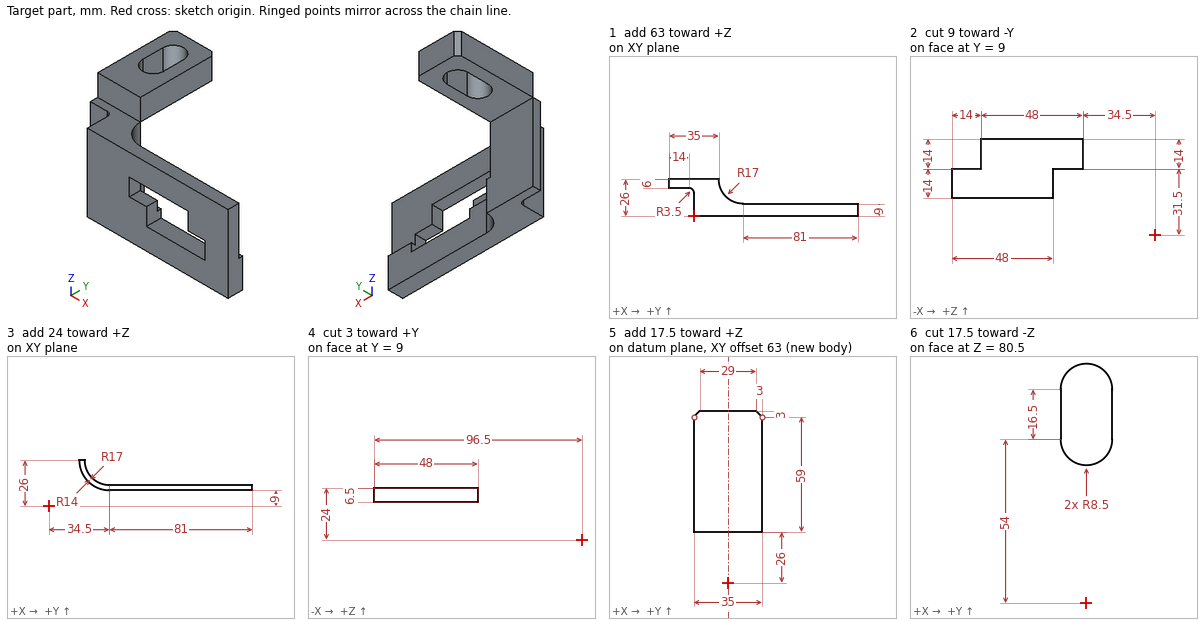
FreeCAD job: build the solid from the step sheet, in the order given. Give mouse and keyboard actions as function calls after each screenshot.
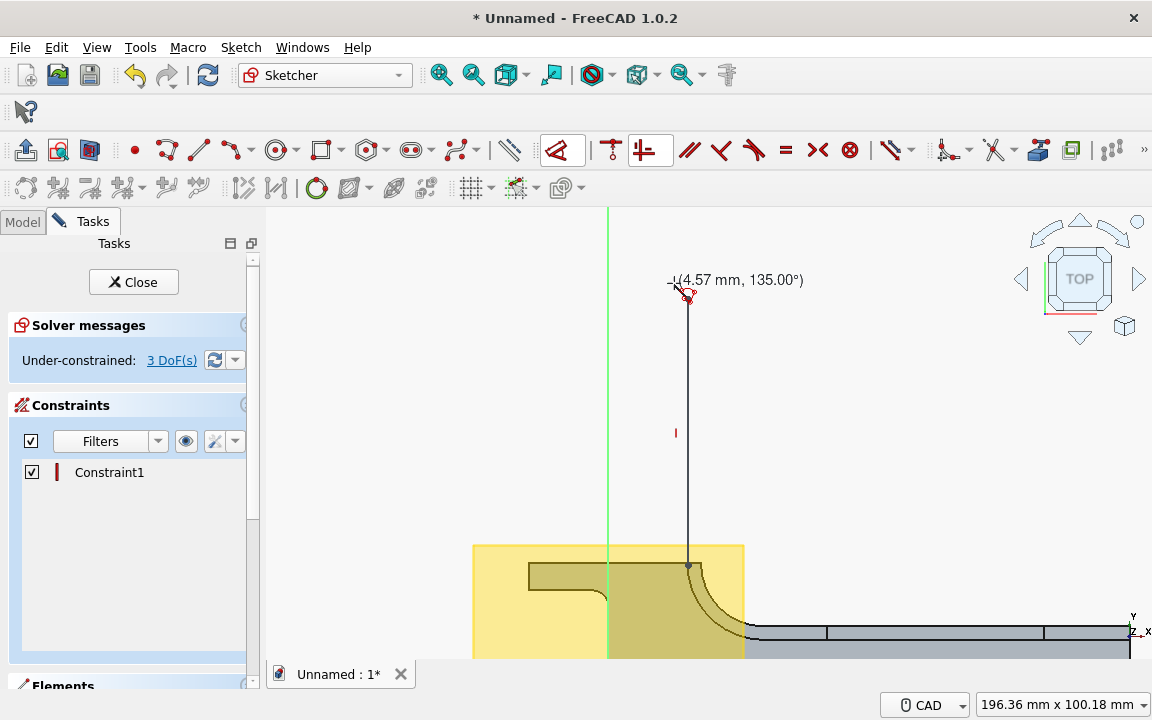
click(674, 283)
click(543, 283)
click(529, 297)
click(529, 563)
click(688, 565)
key(Escape)
key(Escape)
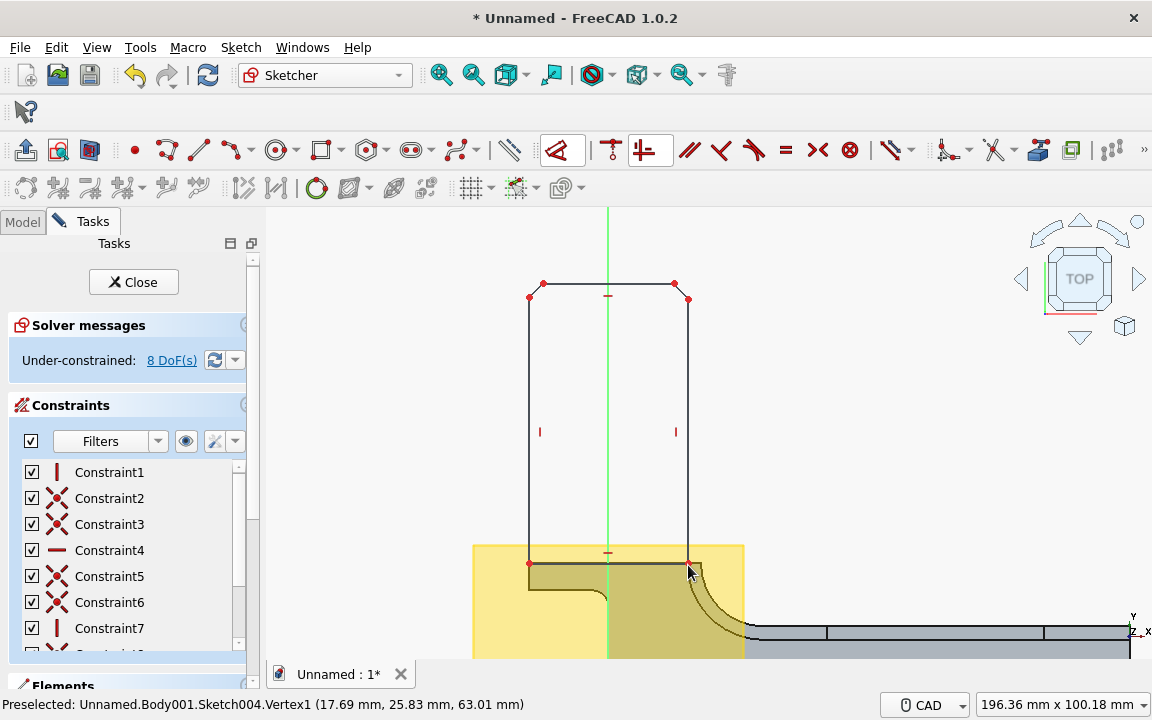
click(688, 299)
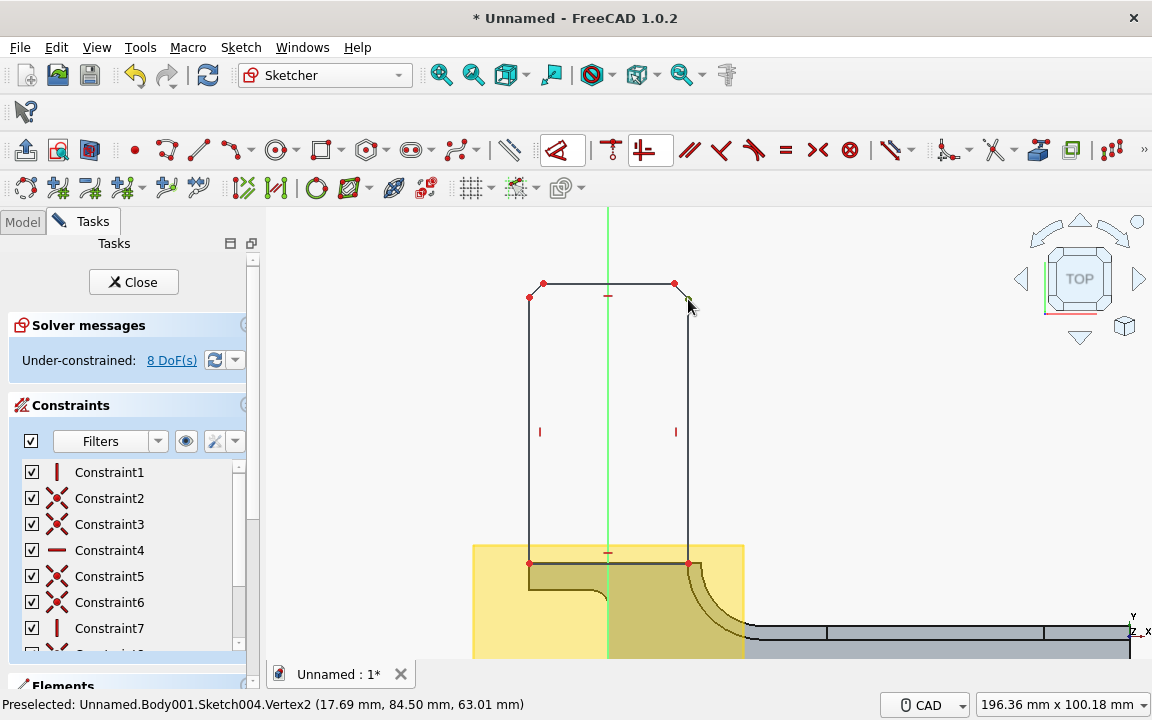
click(529, 298)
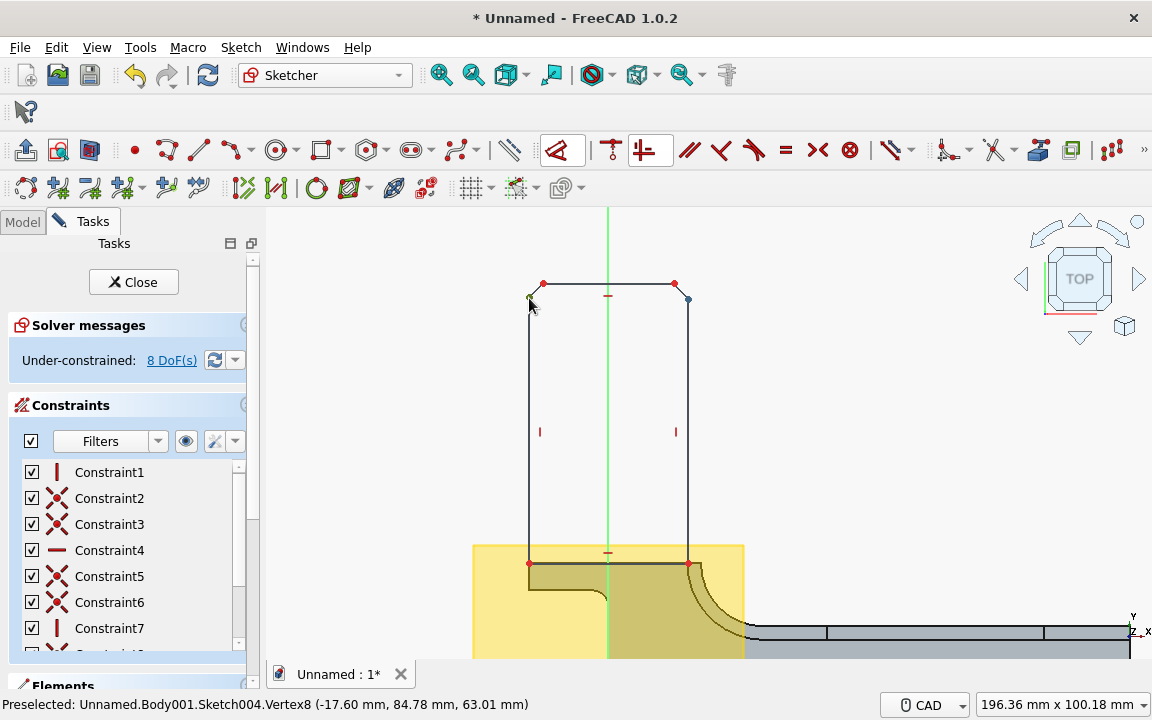
click(608, 603)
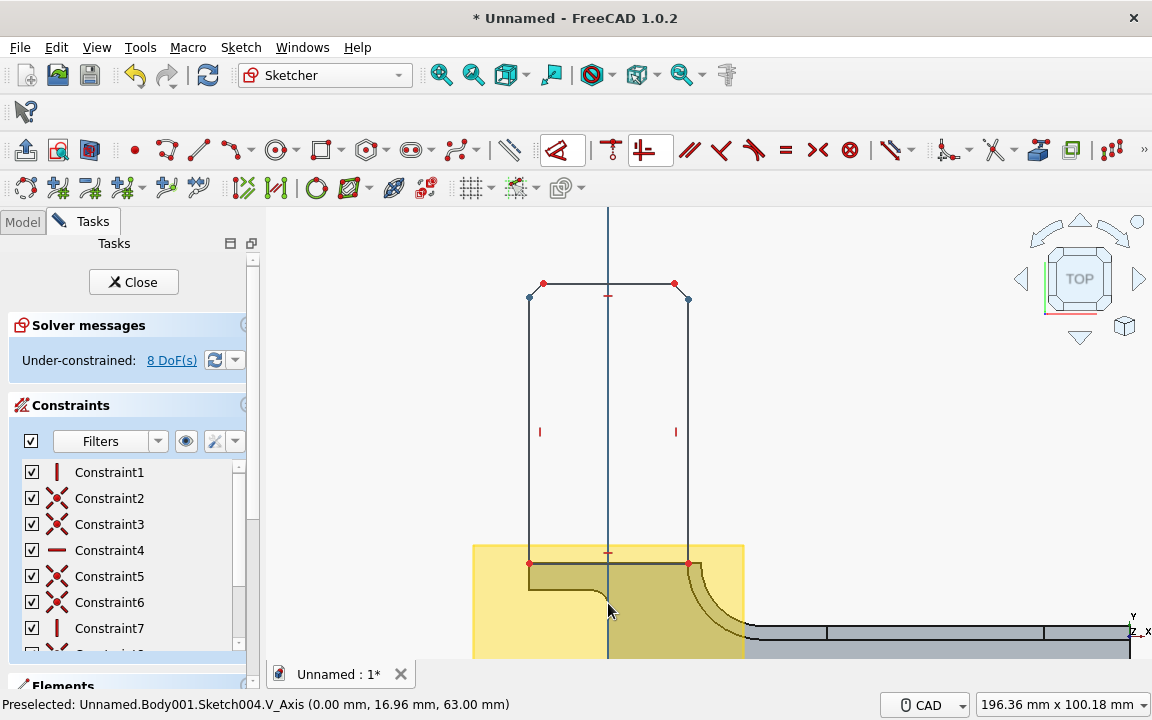
key(s)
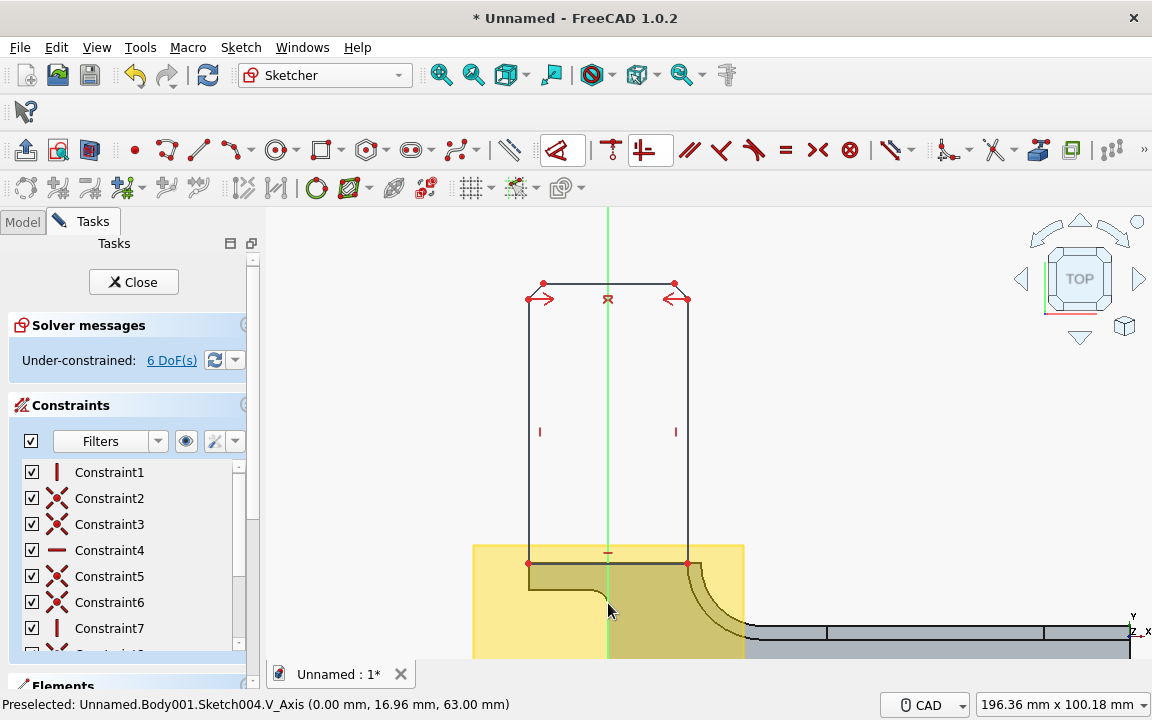
click(688, 485)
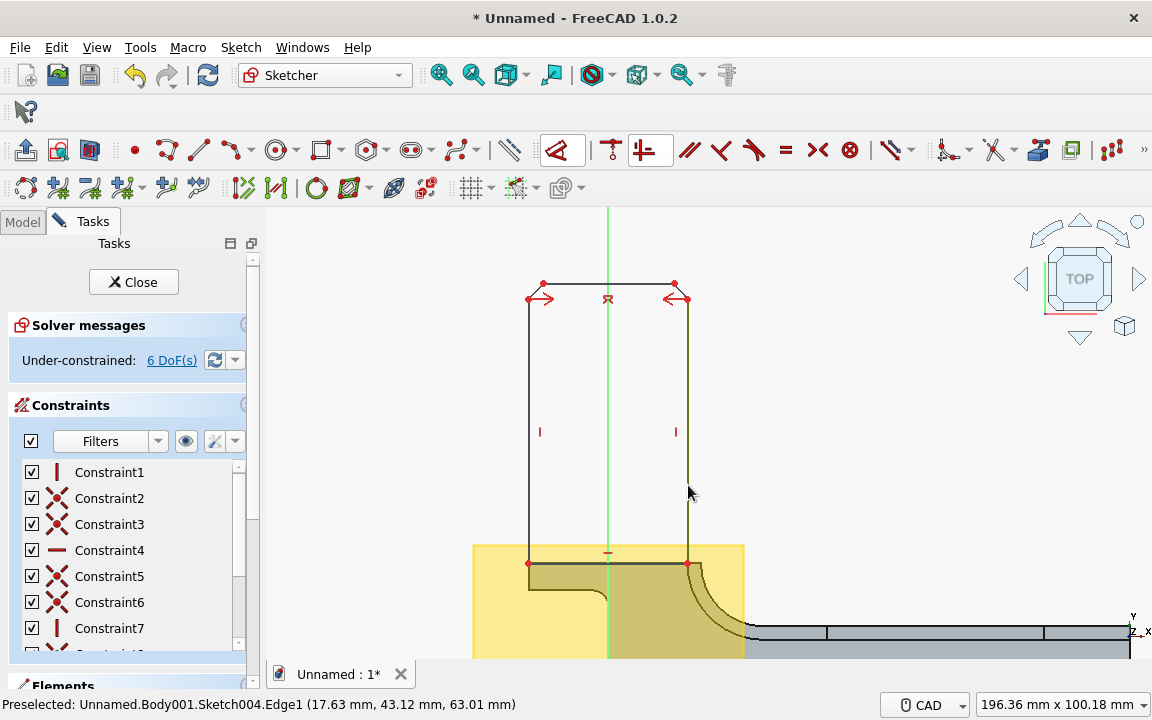
key(i)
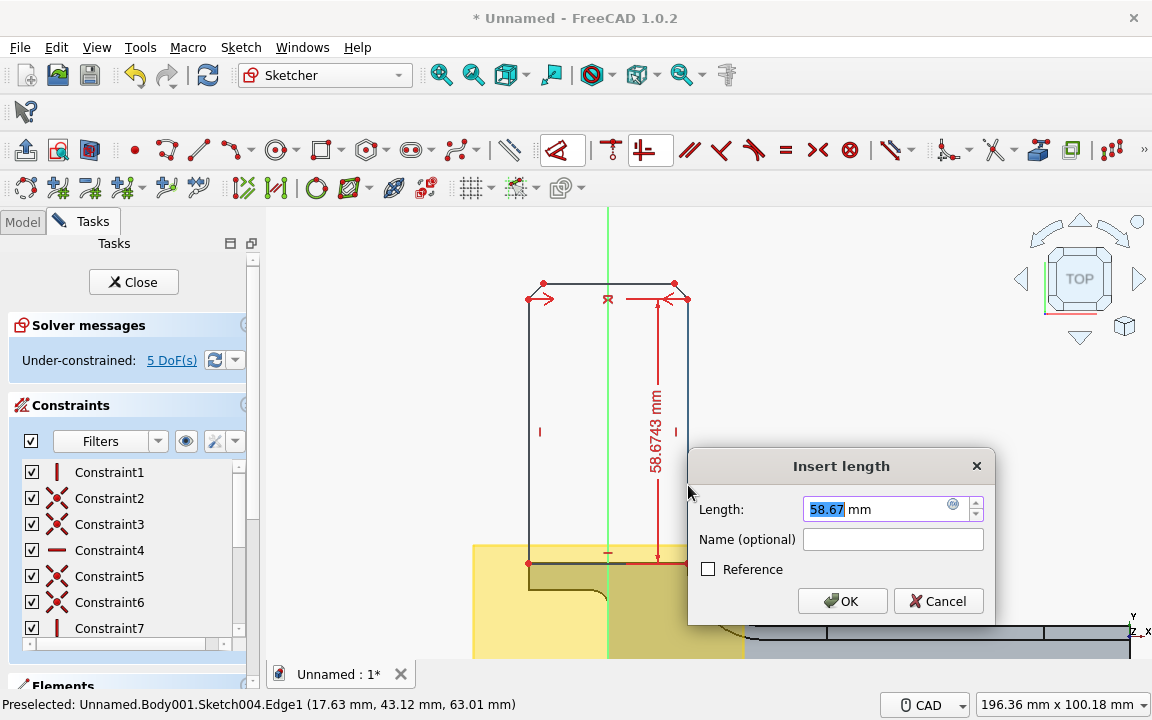
text(59)
key(Return)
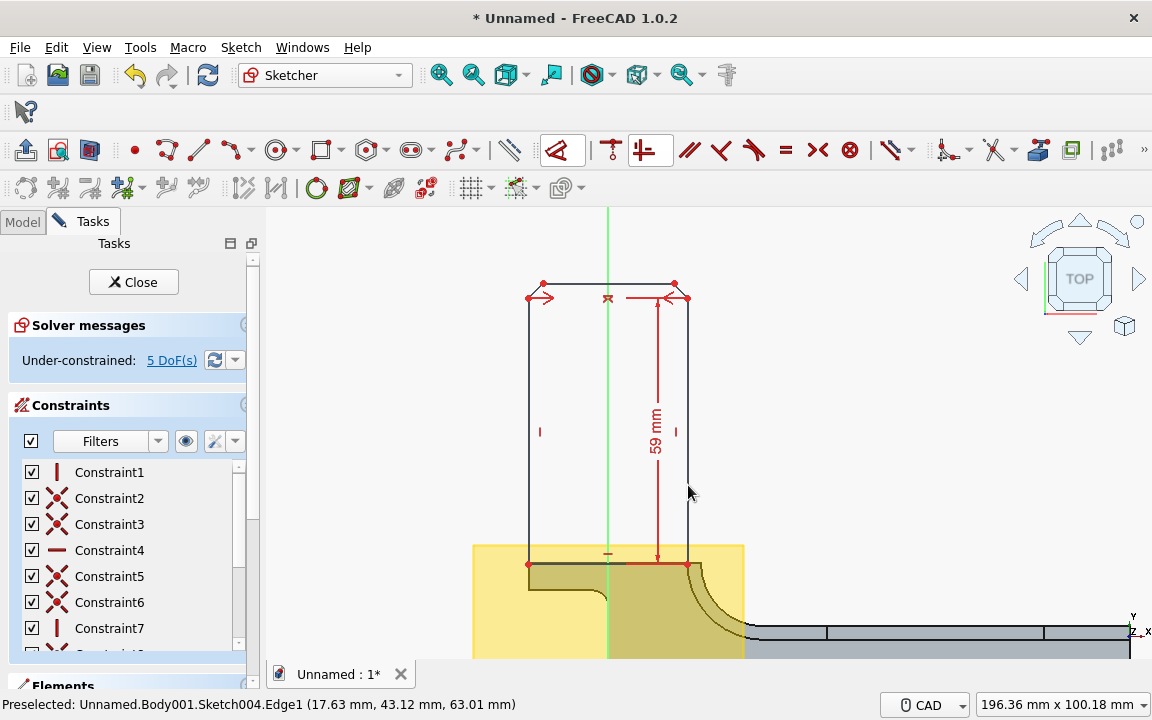
click(635, 284)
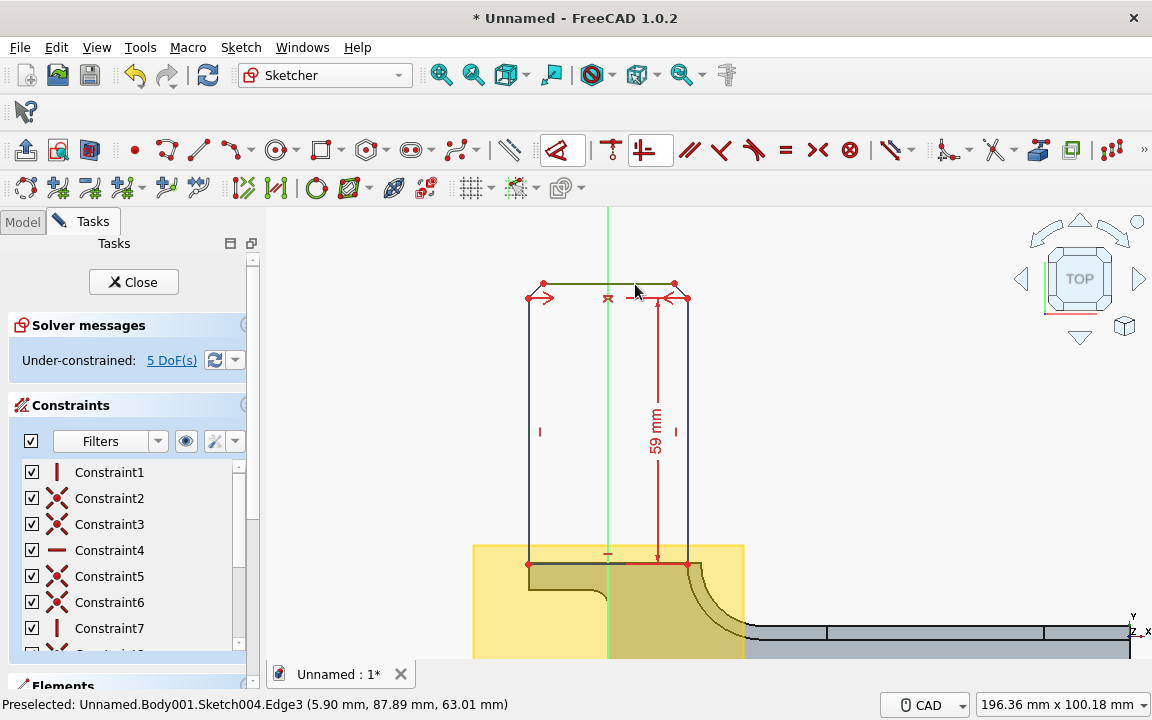
key(l)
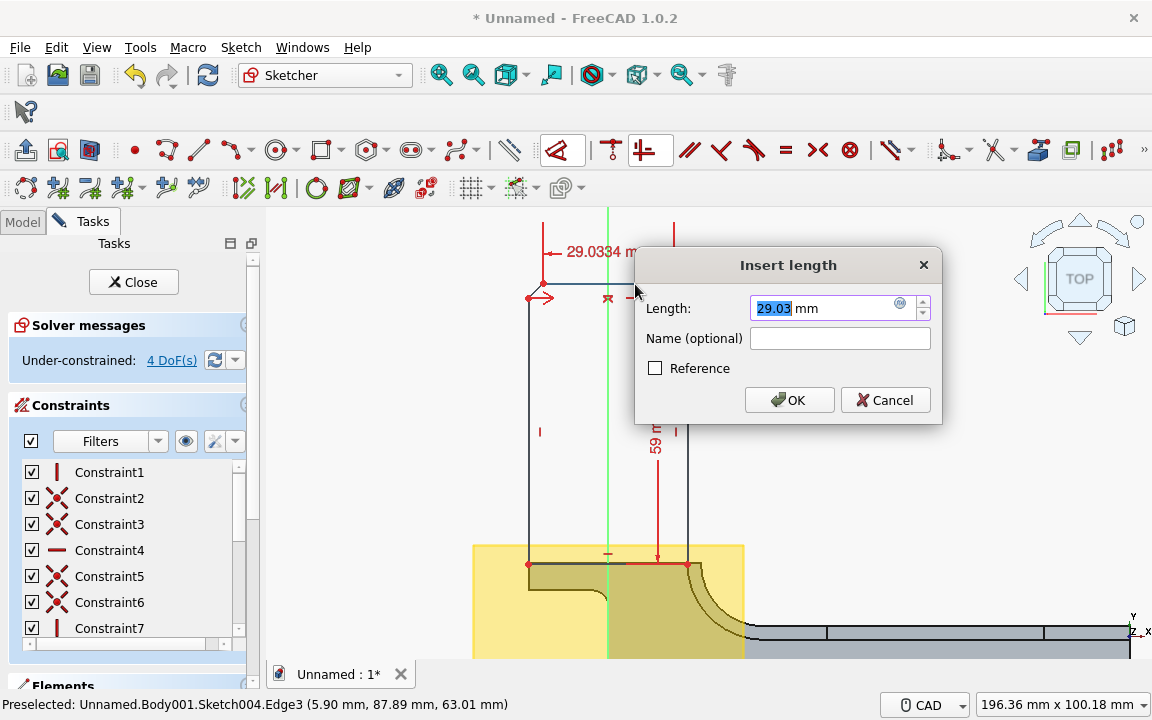
text(29)
key(Return)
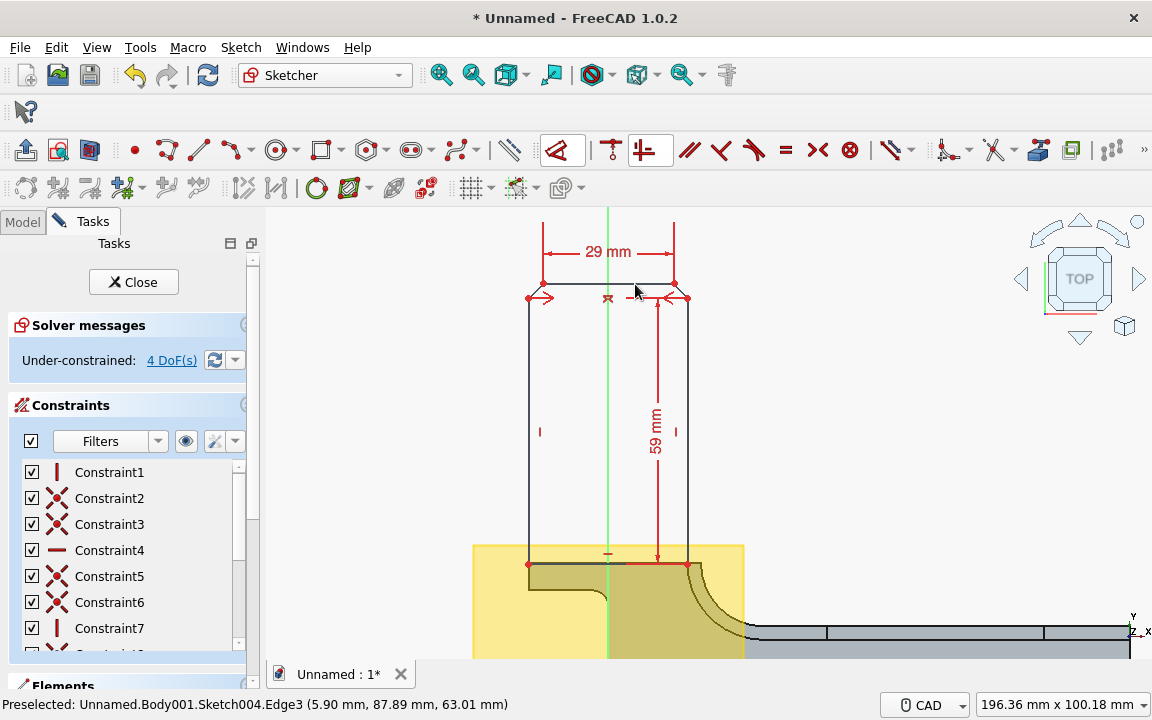
click(577, 564)